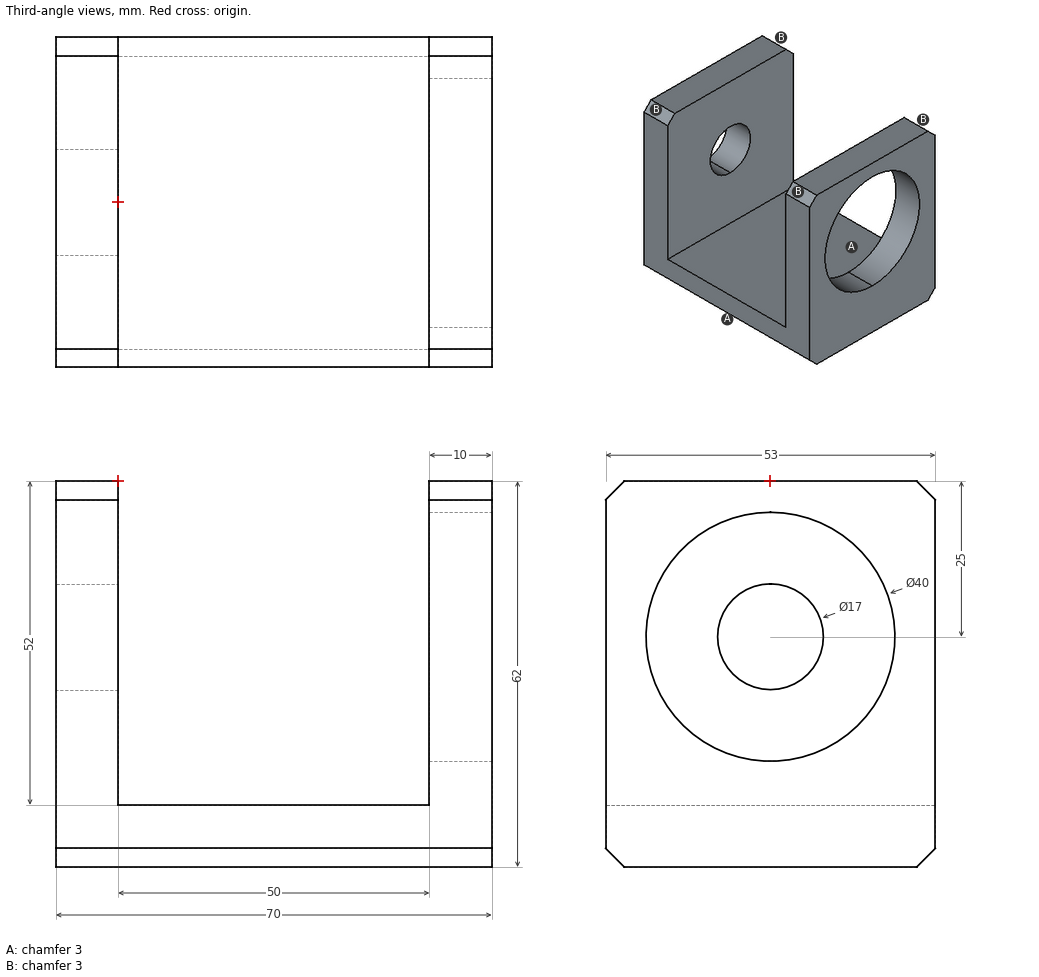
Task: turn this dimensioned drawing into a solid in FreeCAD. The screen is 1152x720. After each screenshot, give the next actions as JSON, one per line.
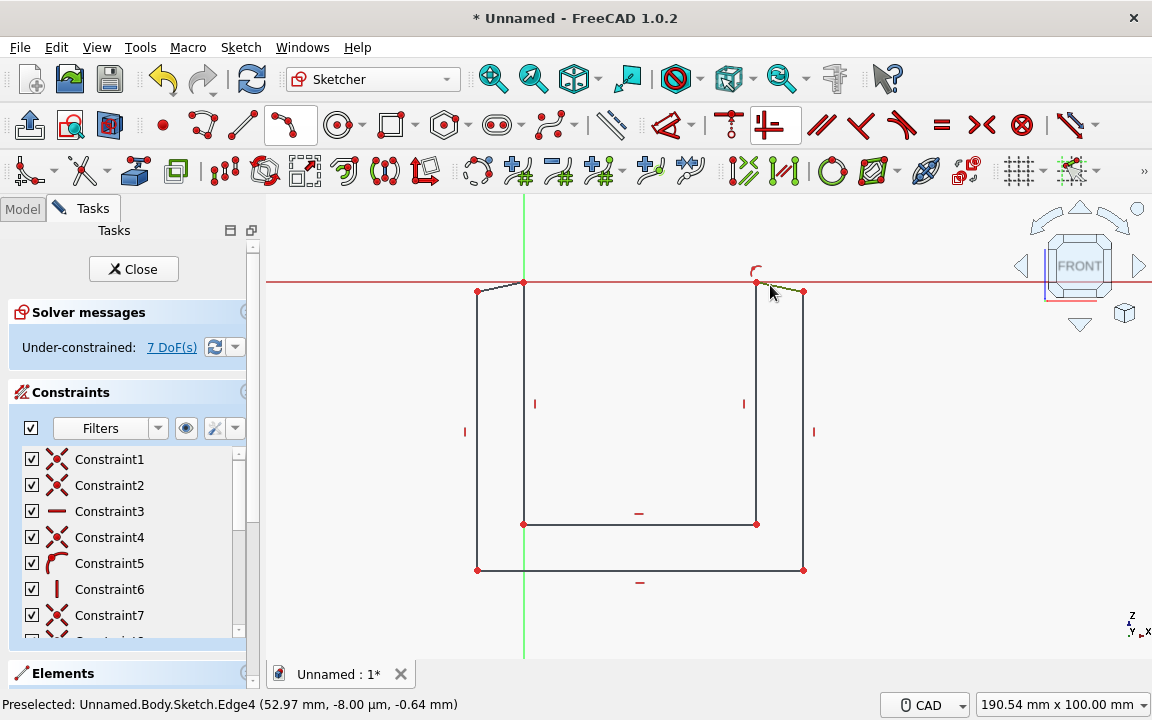
{"action": "key", "text": "h"}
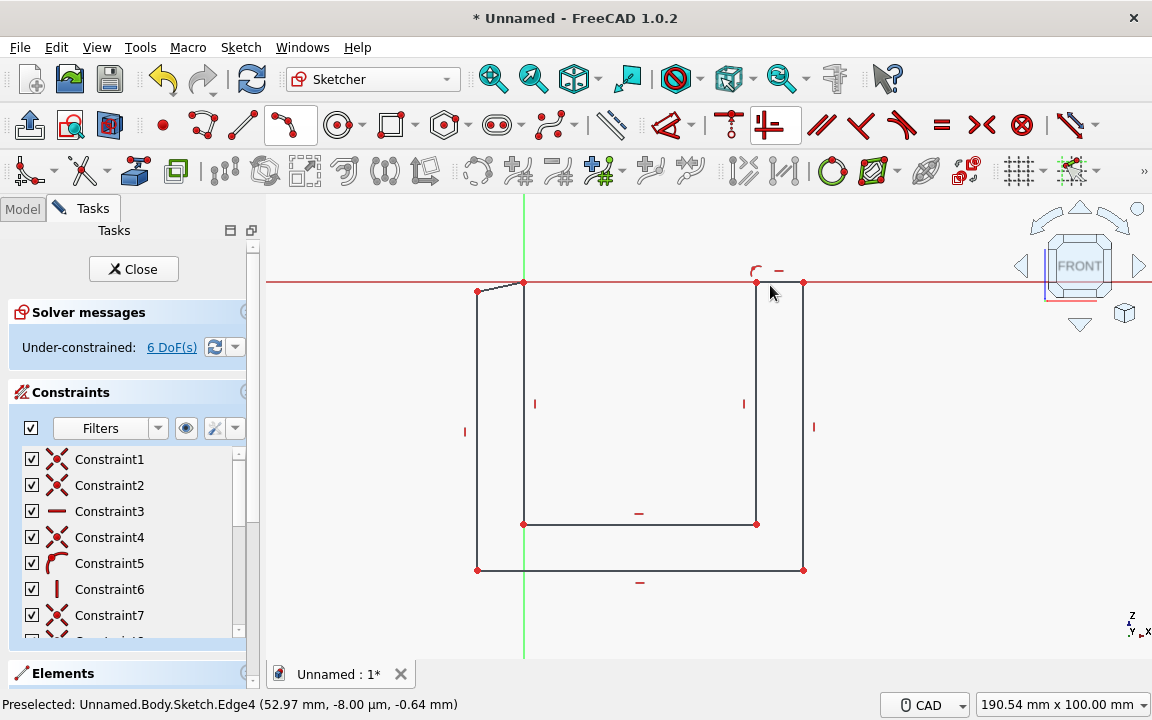
{"action": "left_click", "coordinate": [510, 285]}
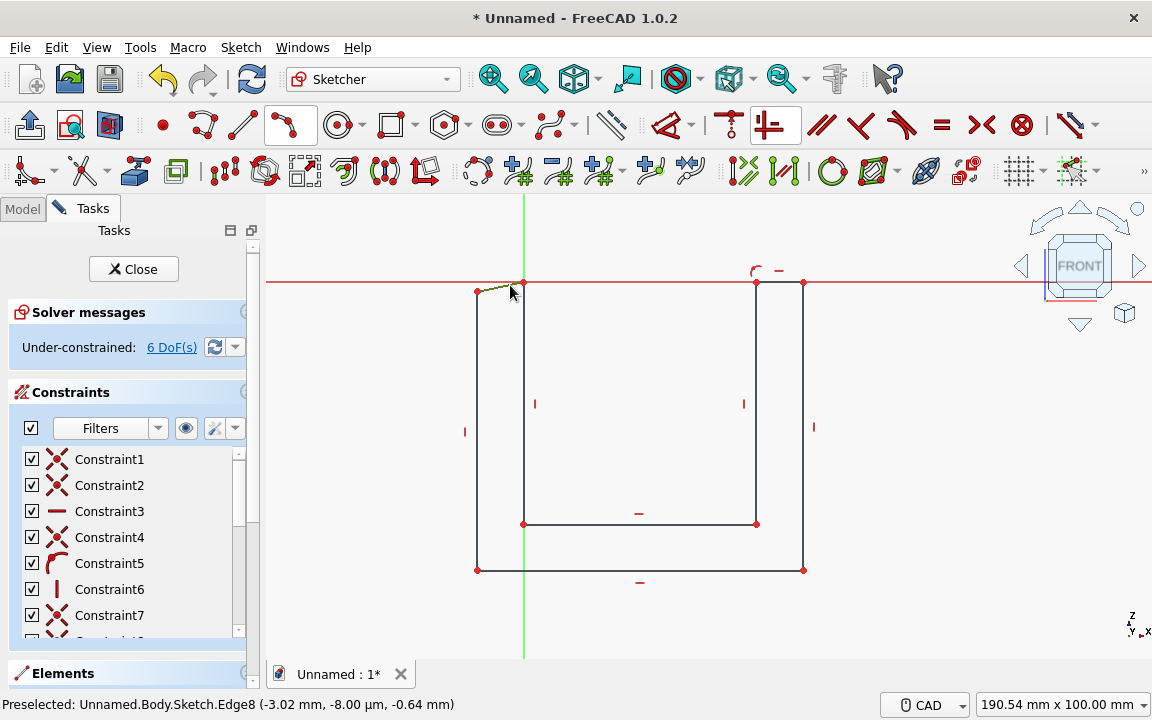
{"action": "key", "text": "h"}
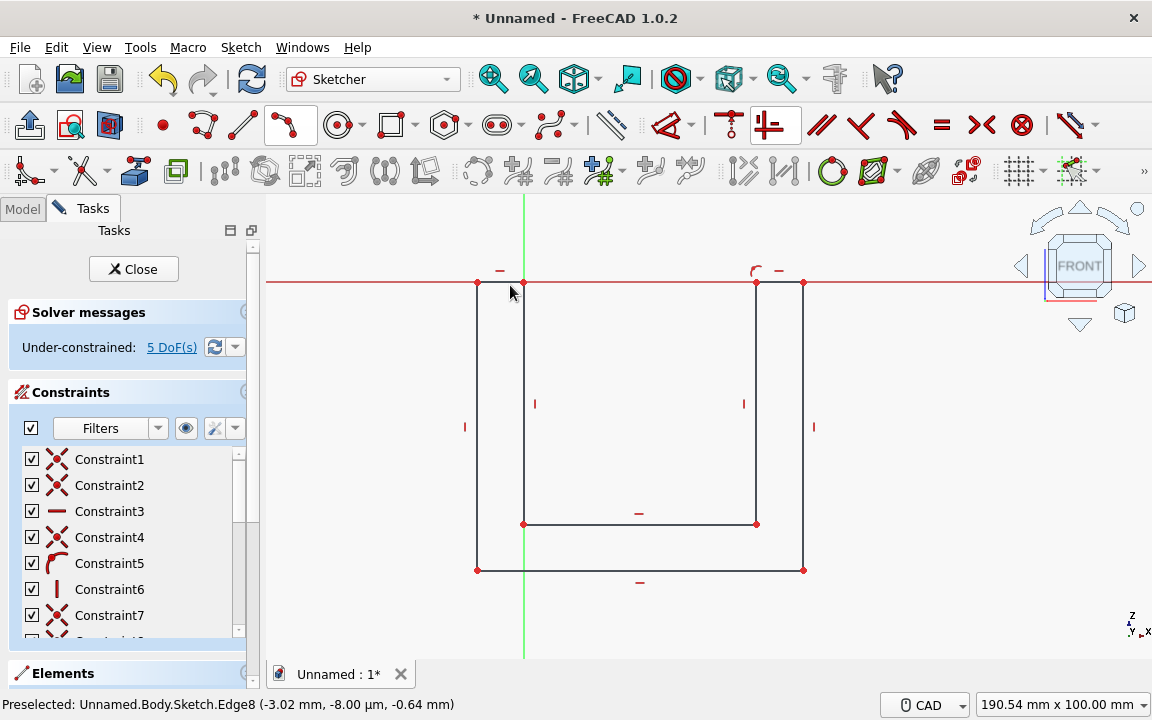
{"action": "key", "text": "d"}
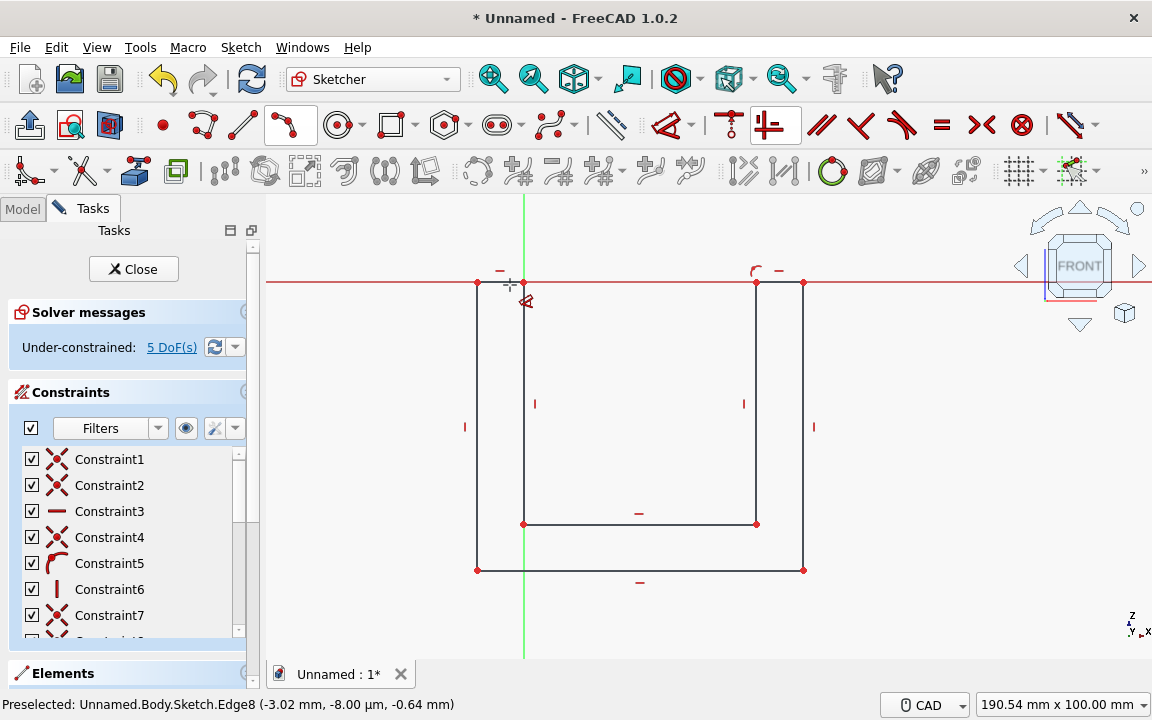
{"action": "left_click", "coordinate": [524, 355]}
{"action": "left_click", "coordinate": [558, 404]}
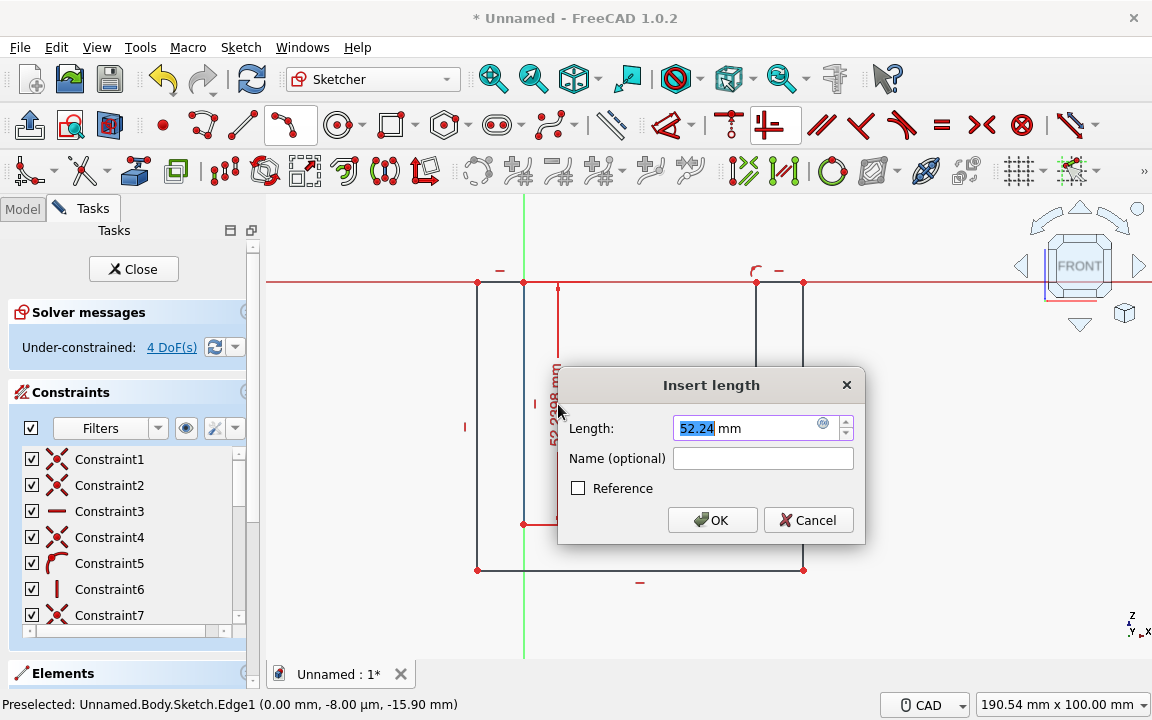
{"action": "type", "text": "52"}
{"action": "key", "text": "Return"}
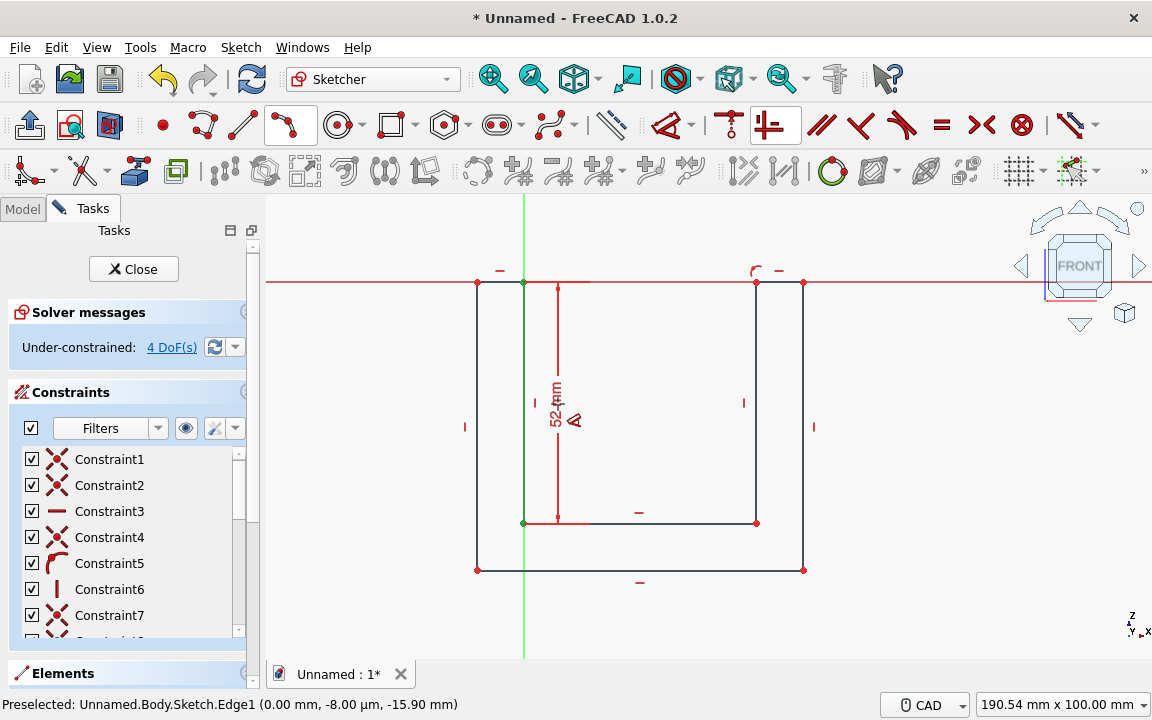
{"action": "left_click", "coordinate": [594, 524]}
{"action": "left_click", "coordinate": [640, 558]}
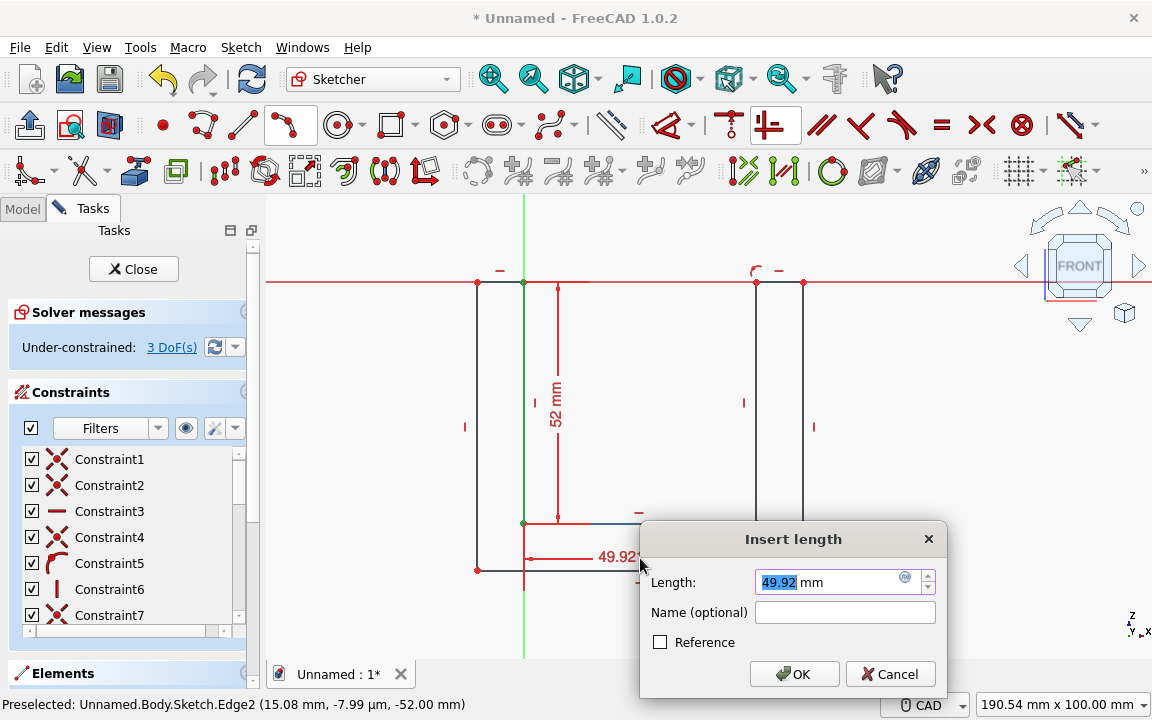
{"action": "type", "text": "50"}
{"action": "key", "text": "Return"}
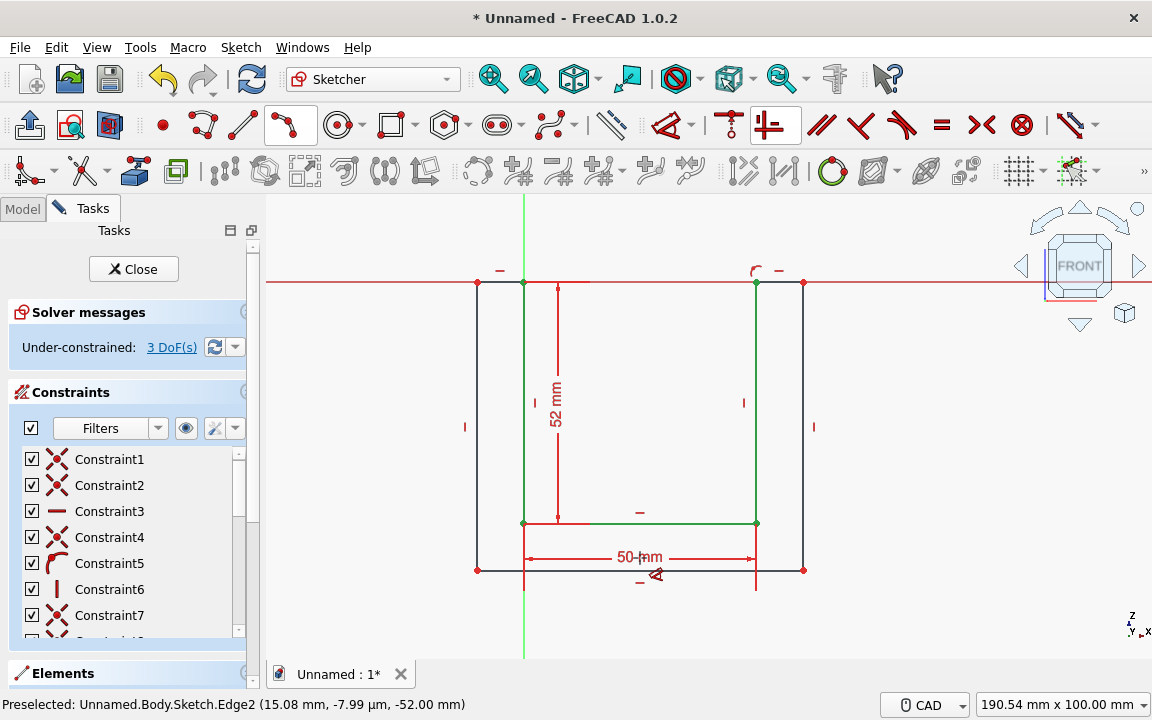
{"action": "left_click", "coordinate": [770, 282]}
{"action": "left_click", "coordinate": [780, 248]}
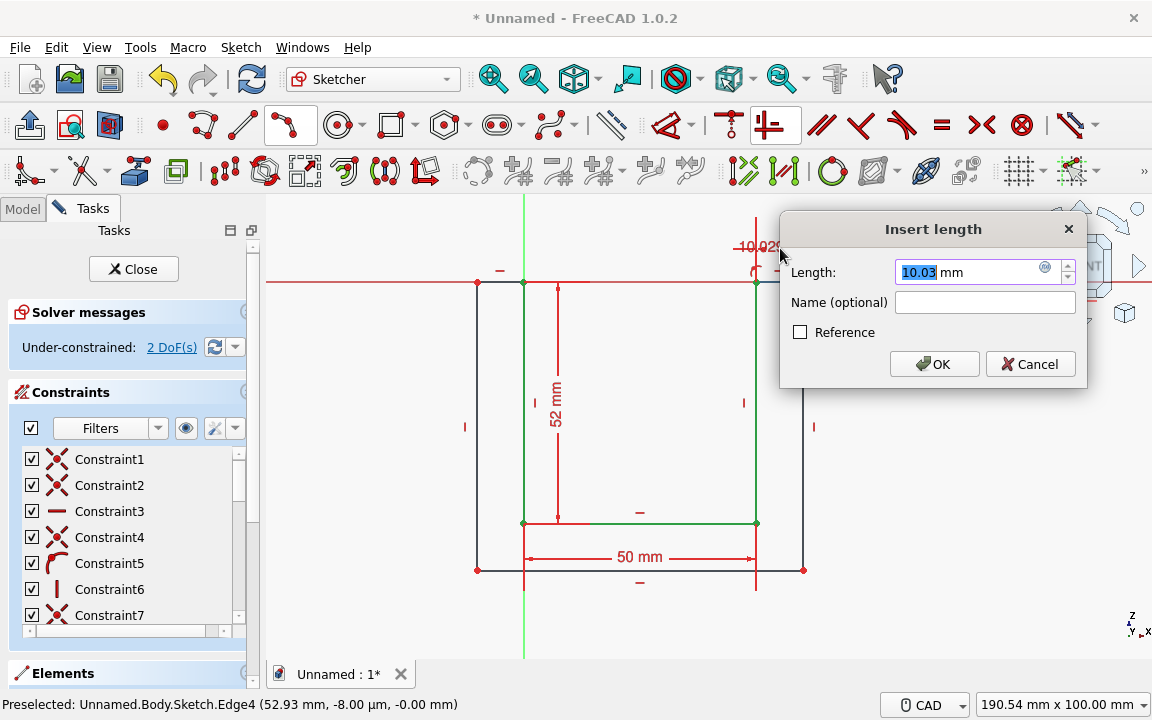
{"action": "type", "text": "10"}
{"action": "key", "text": "Return"}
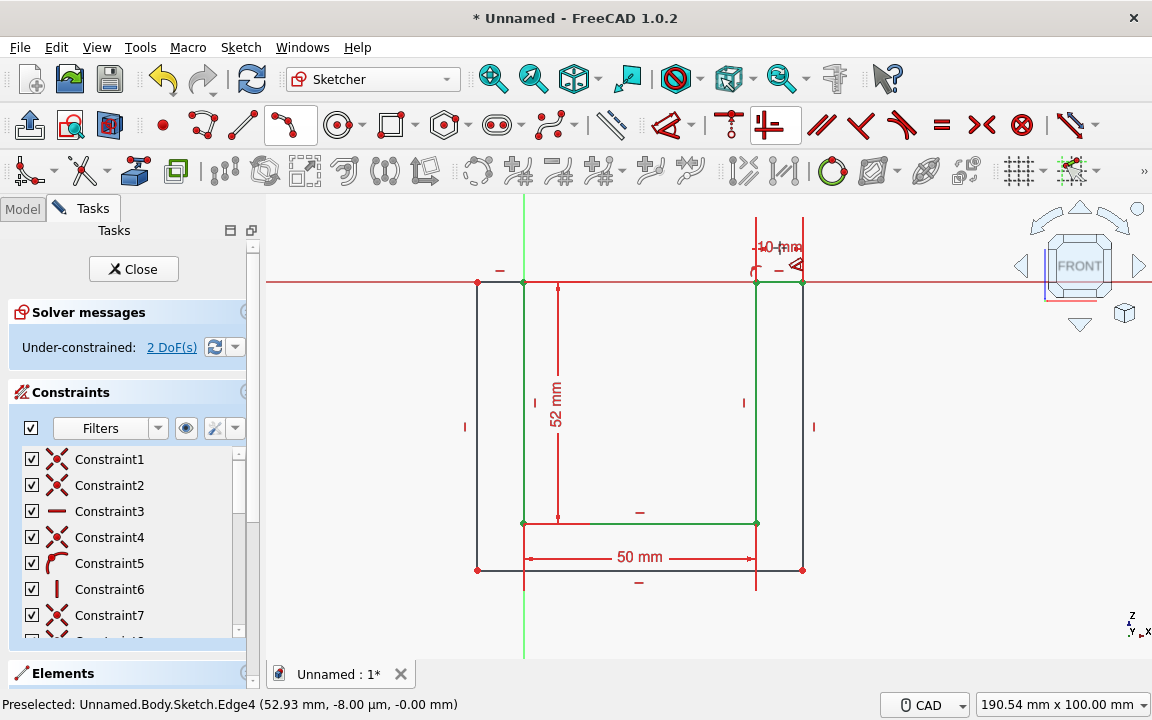
{"action": "left_click", "coordinate": [803, 369]}
{"action": "left_click", "coordinate": [837, 427]}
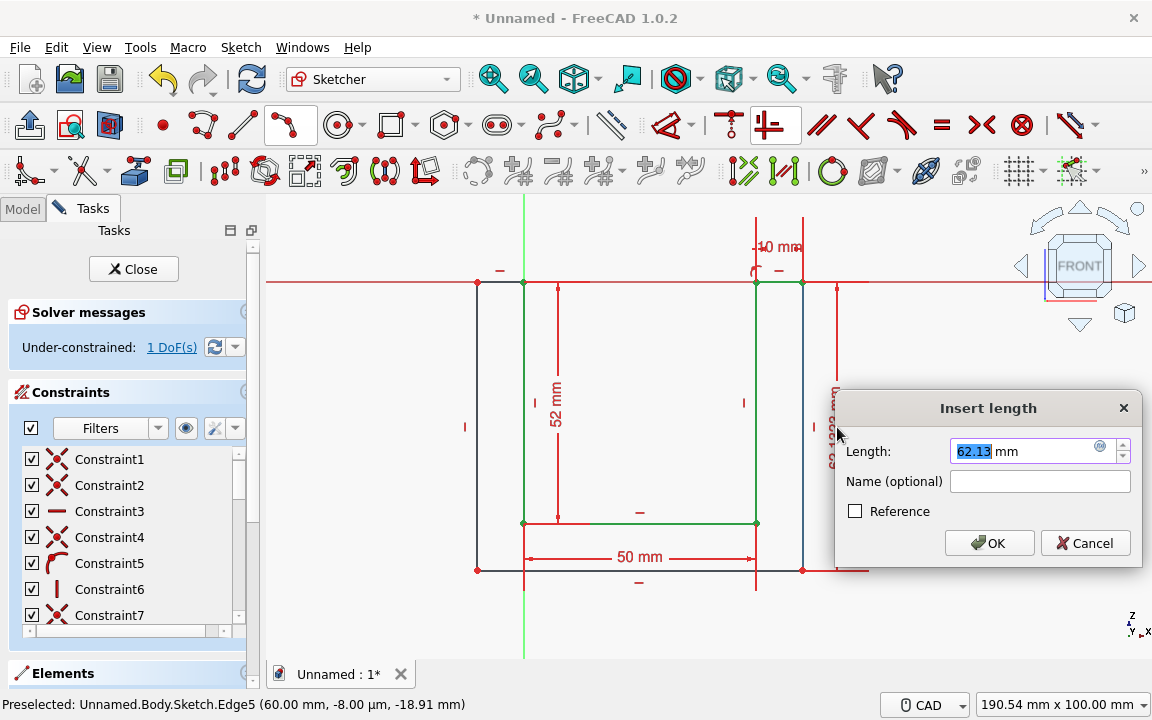
{"action": "type", "text": "62"}
{"action": "key", "text": "Return"}